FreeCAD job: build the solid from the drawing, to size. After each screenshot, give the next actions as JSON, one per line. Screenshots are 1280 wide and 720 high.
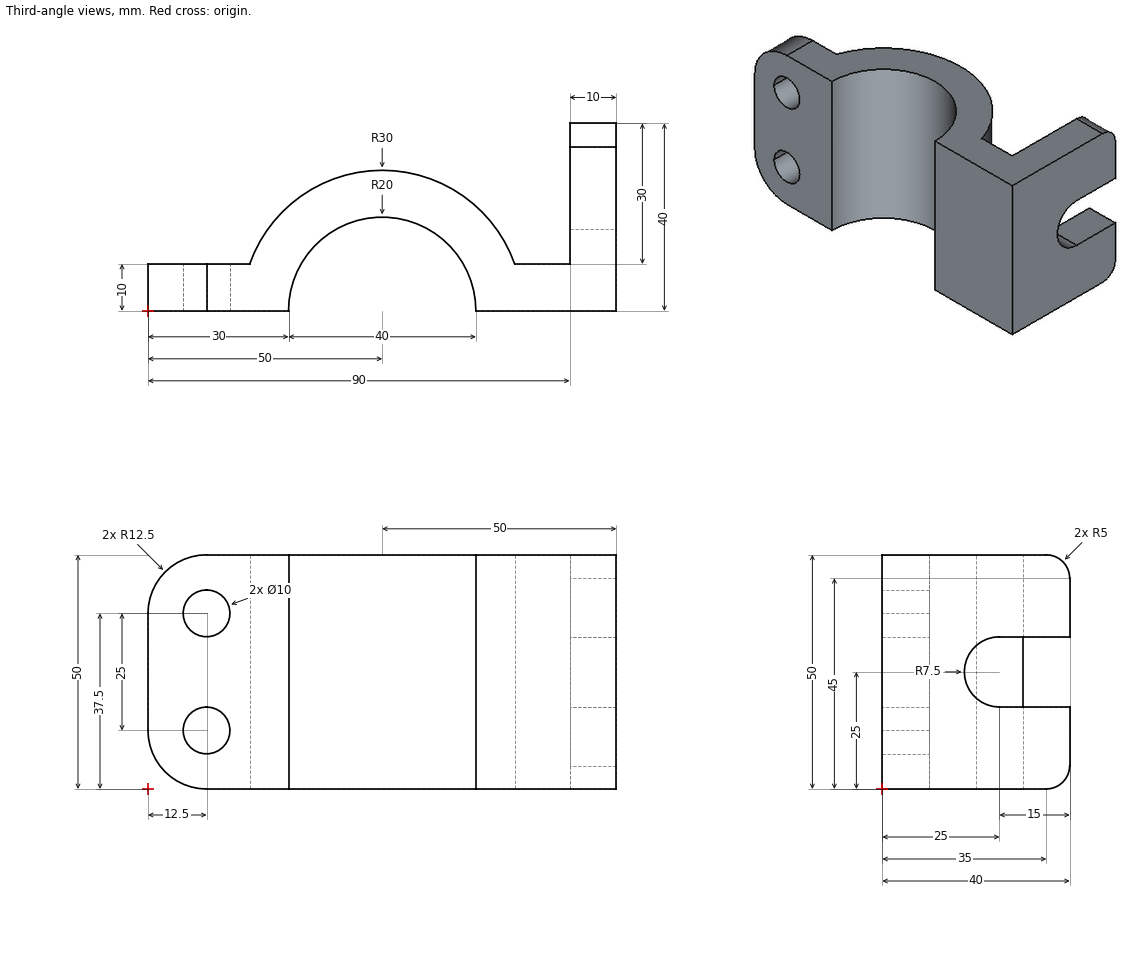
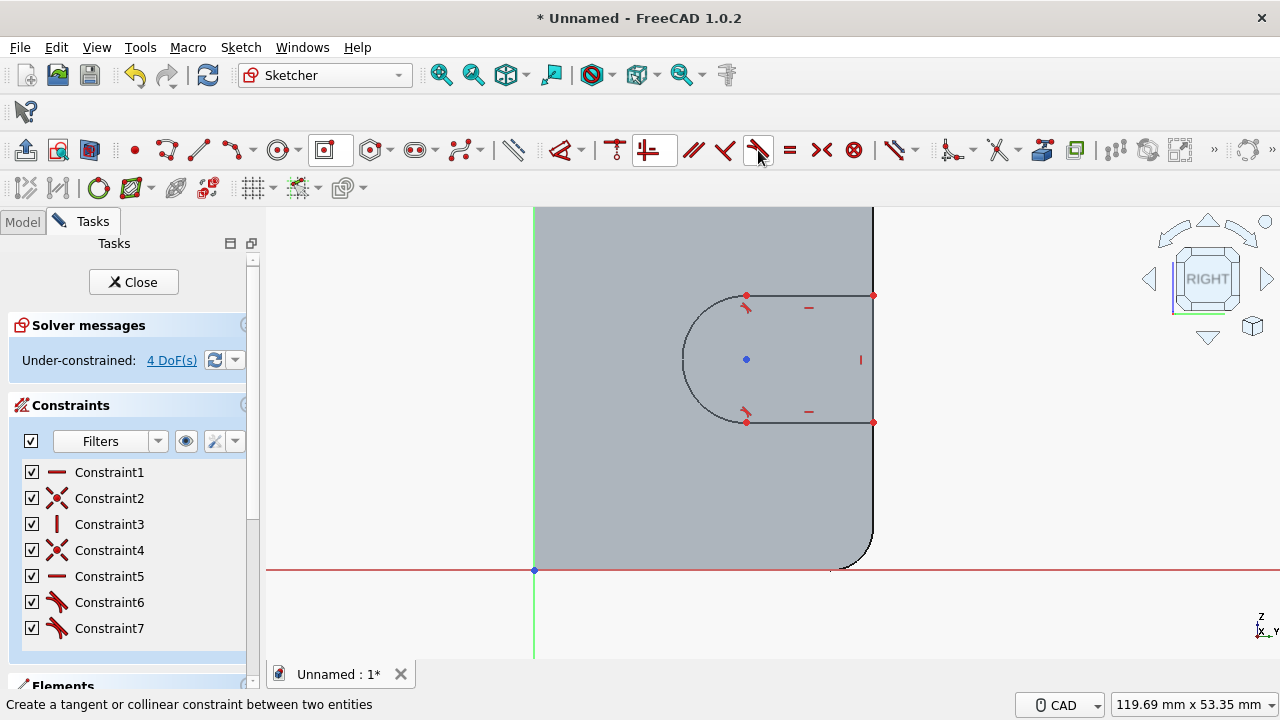
{"action": "left_click", "coordinate": [560, 150]}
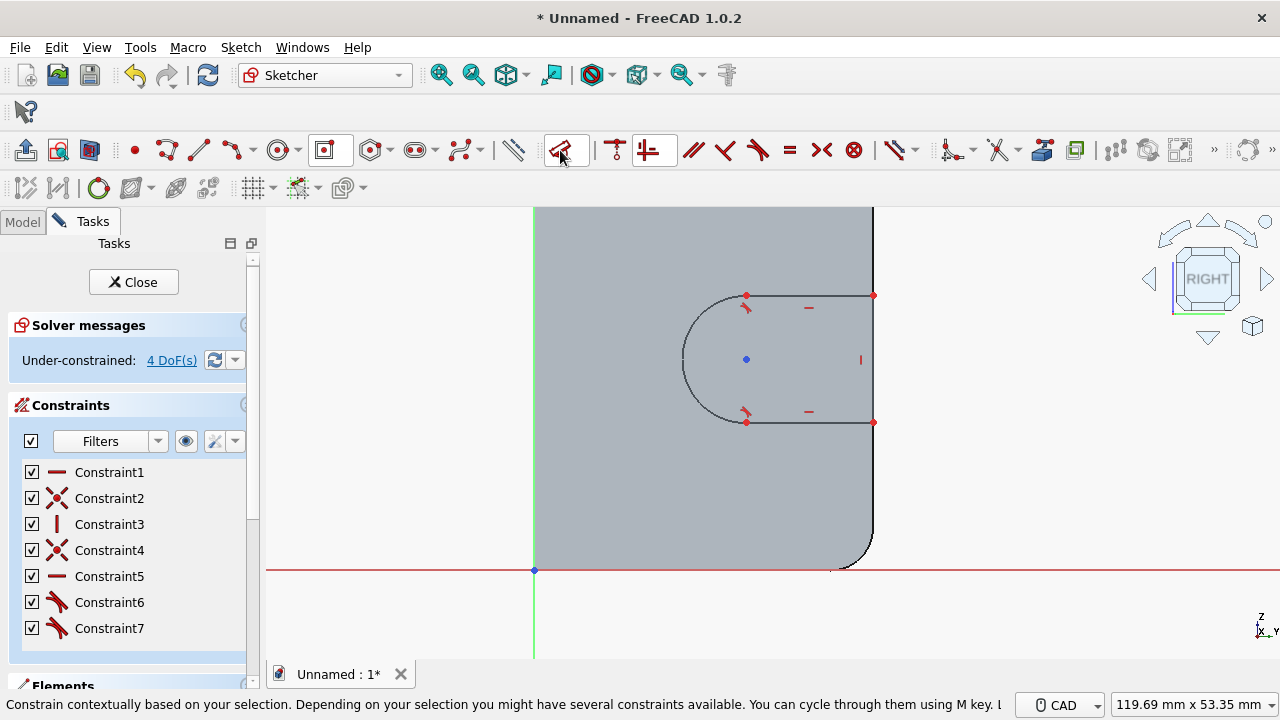
{"action": "left_click", "coordinate": [695, 322]}
{"action": "left_click", "coordinate": [669, 303]}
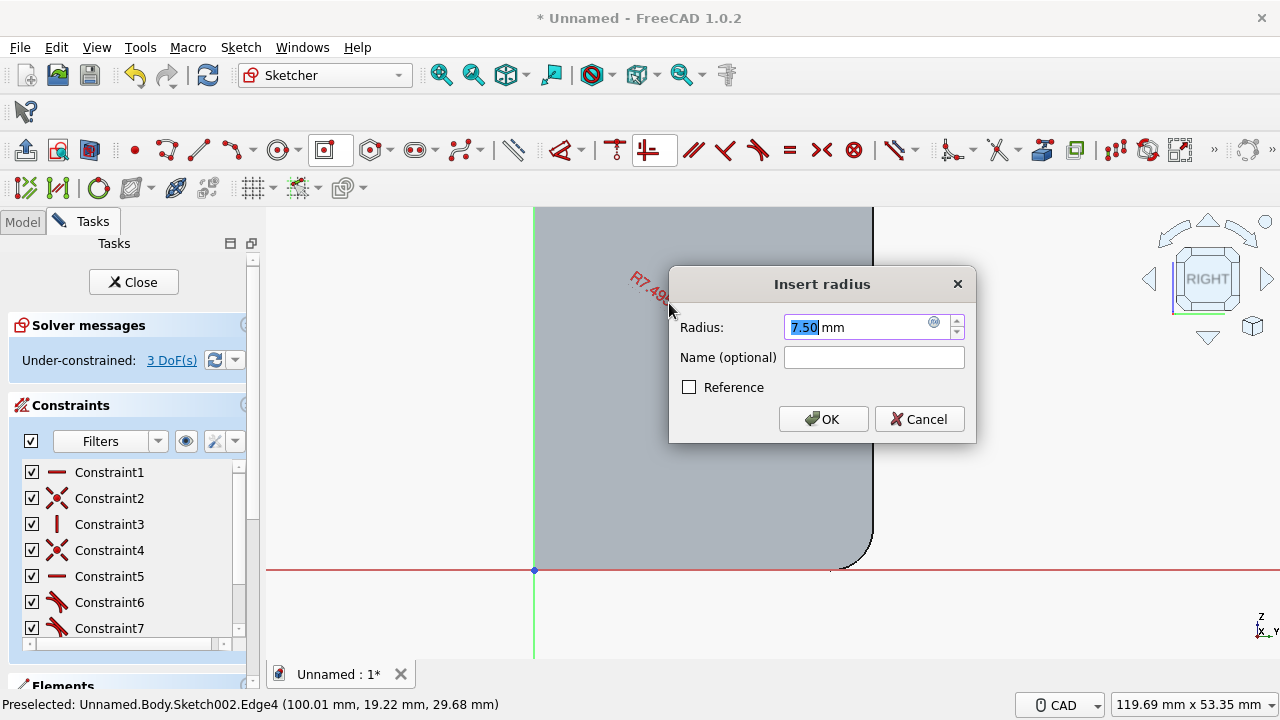
{"action": "type", "text": "7.5"}
{"action": "key", "text": "Return"}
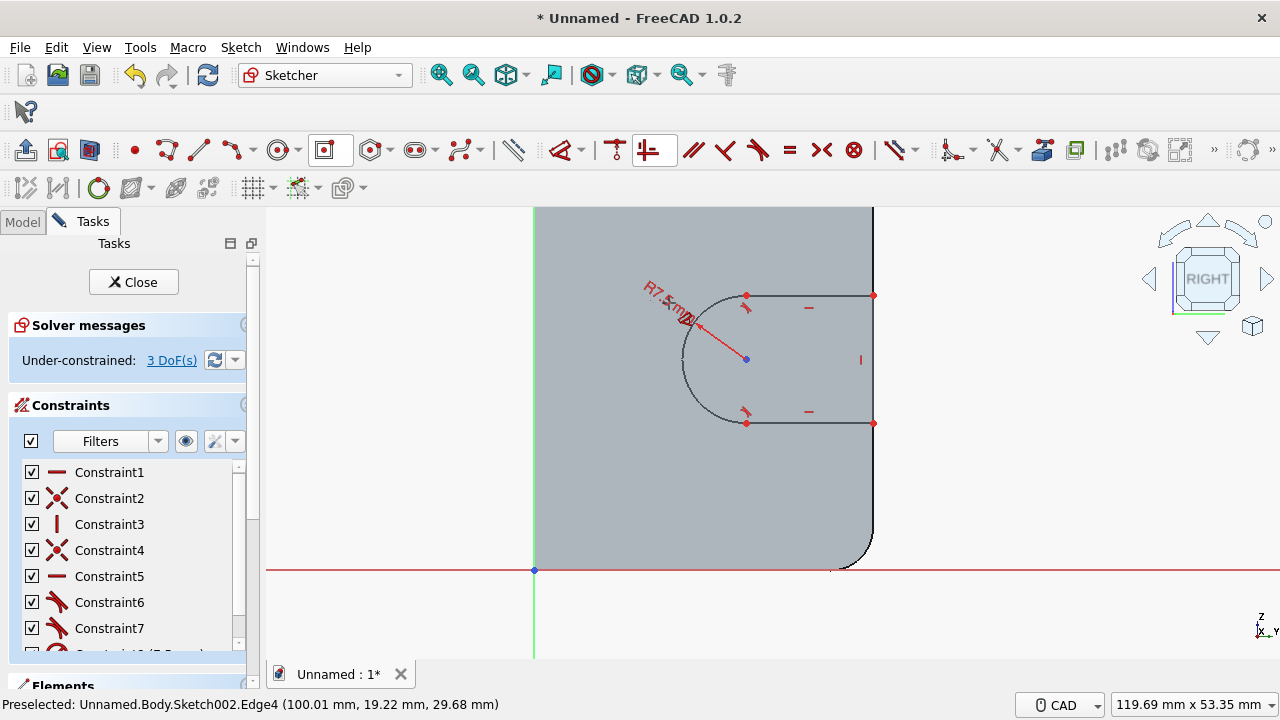
{"action": "left_click", "coordinate": [784, 423]}
{"action": "left_click", "coordinate": [810, 389]}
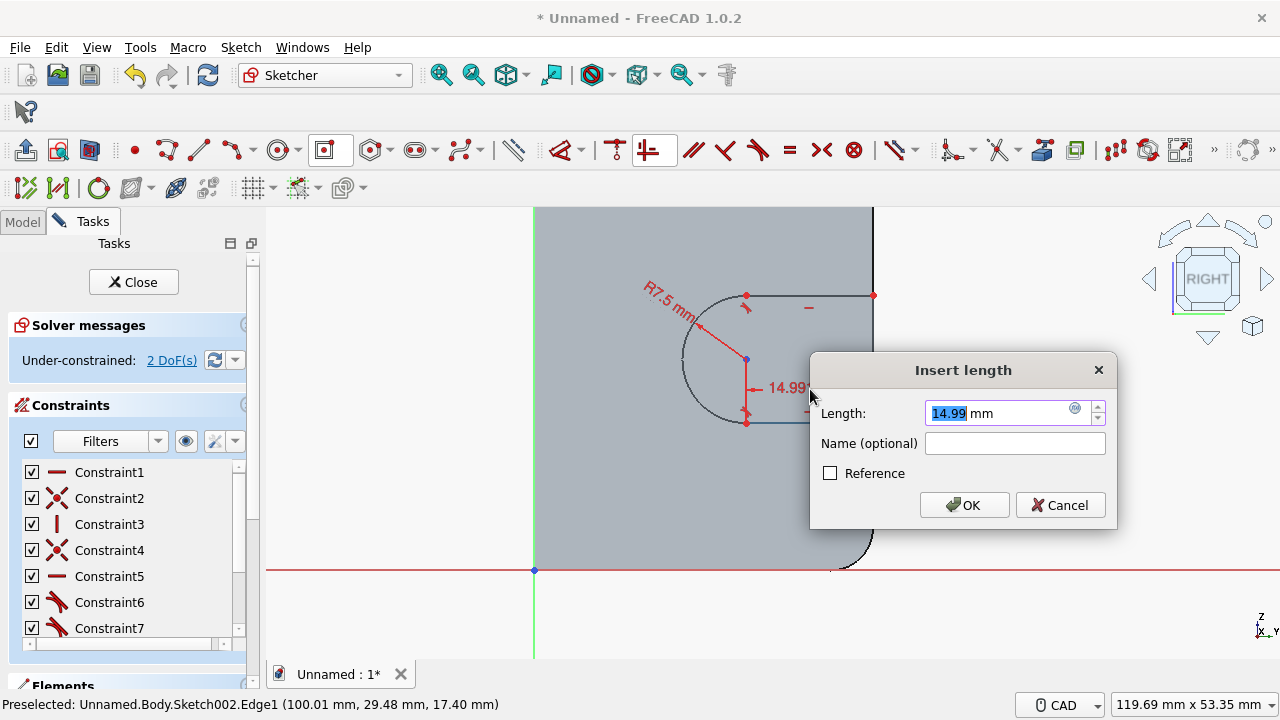
{"action": "type", "text": "15"}
{"action": "key", "text": "Return"}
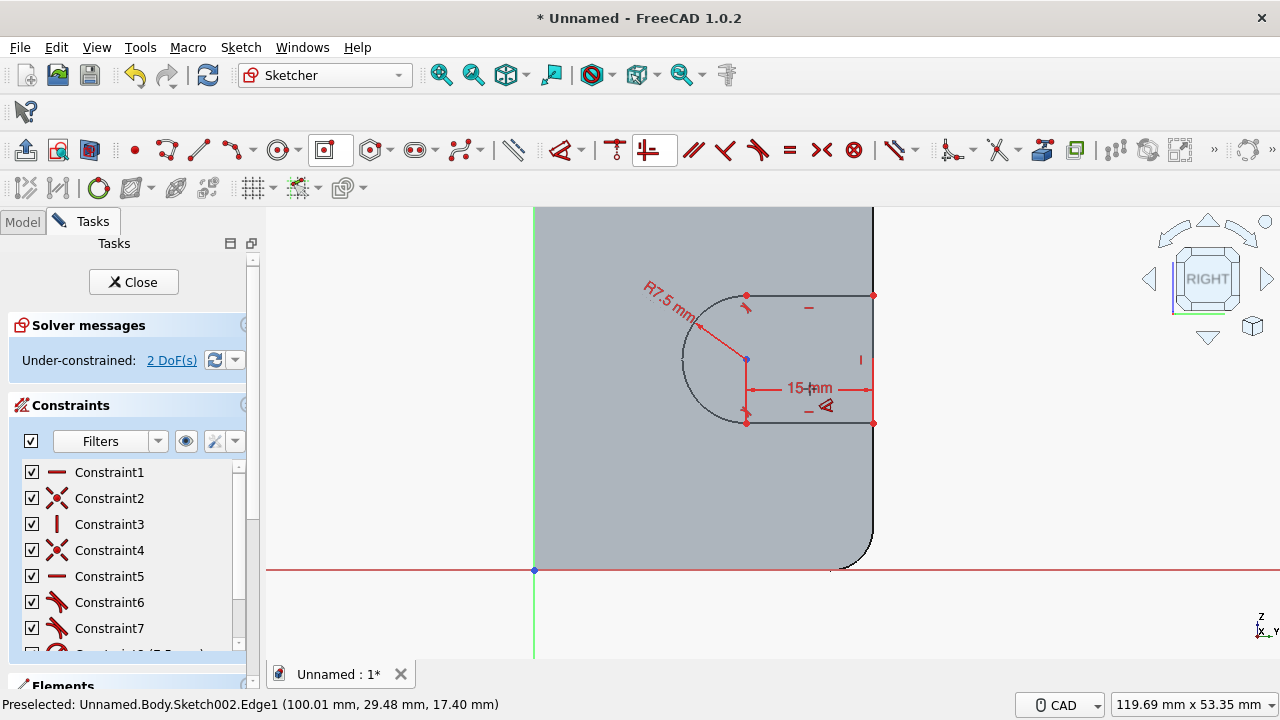
{"action": "left_click", "coordinate": [746, 423]}
{"action": "left_click", "coordinate": [640, 604]}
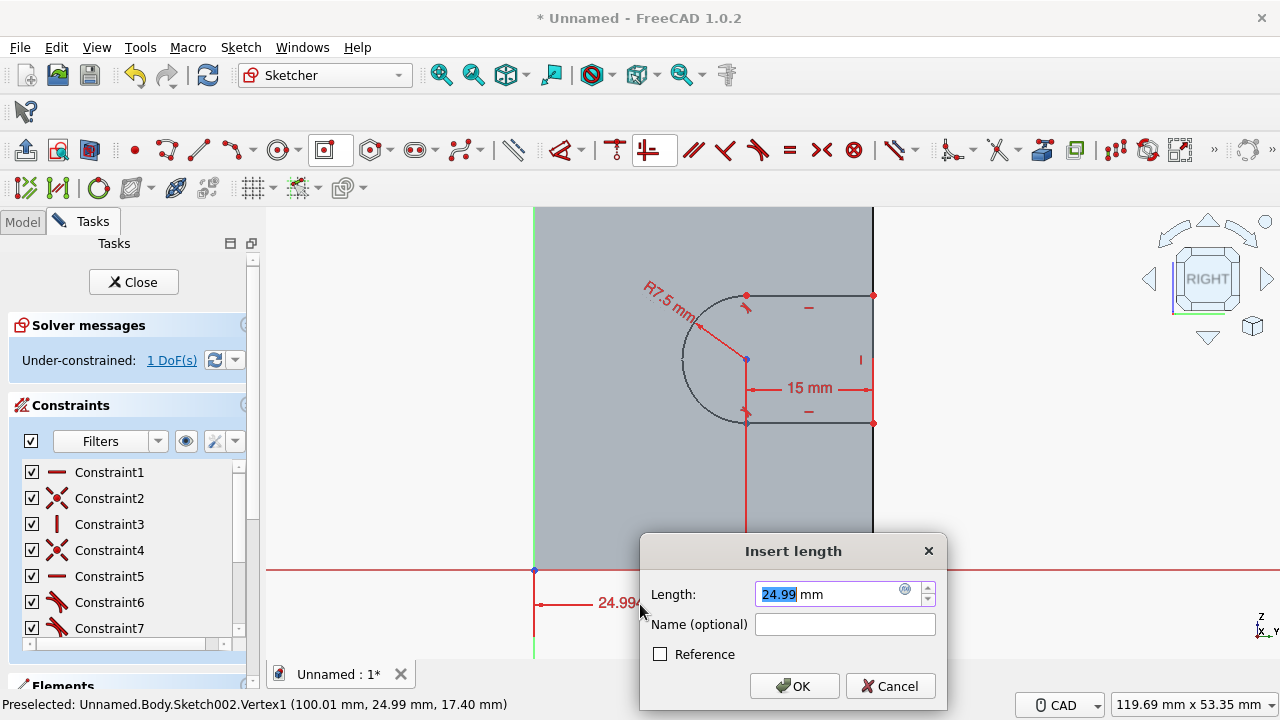
{"action": "type", "text": "25"}
{"action": "key", "text": "Return"}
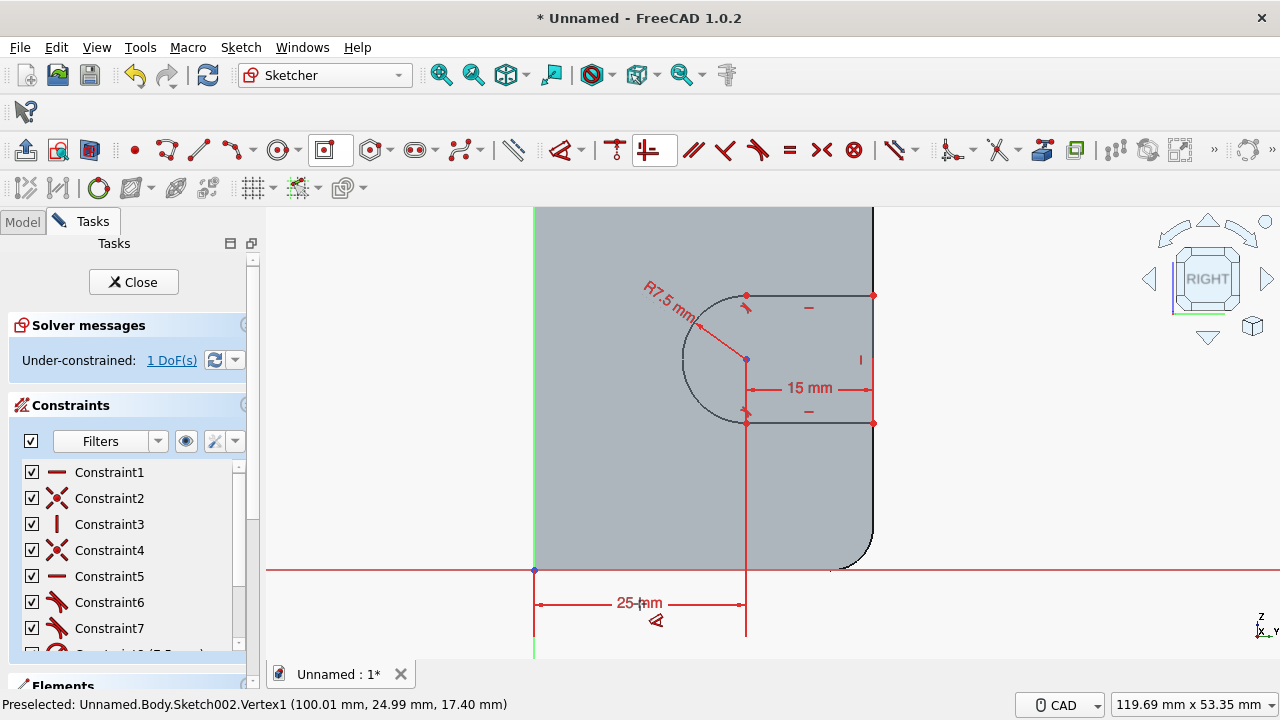
{"action": "left_click", "coordinate": [746, 360]}
{"action": "left_click", "coordinate": [500, 465]}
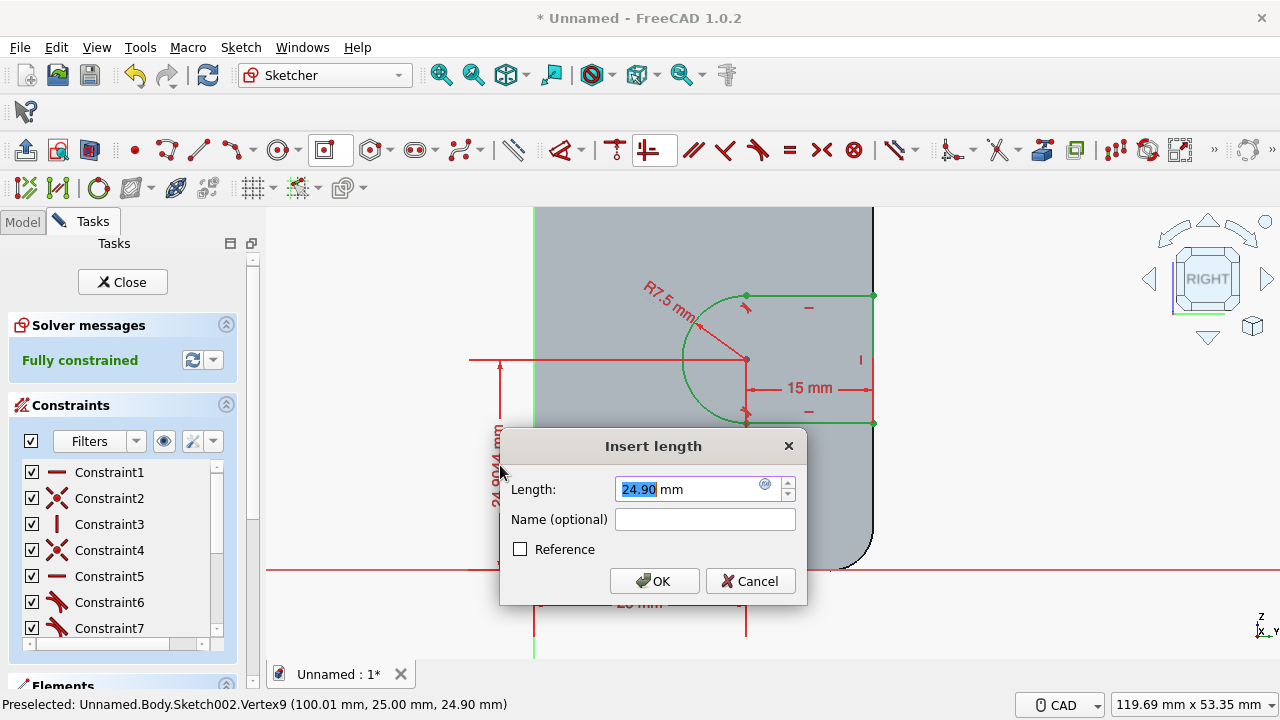
{"action": "type", "text": "25"}
{"action": "key", "text": "Return"}
{"action": "key", "text": "Escape"}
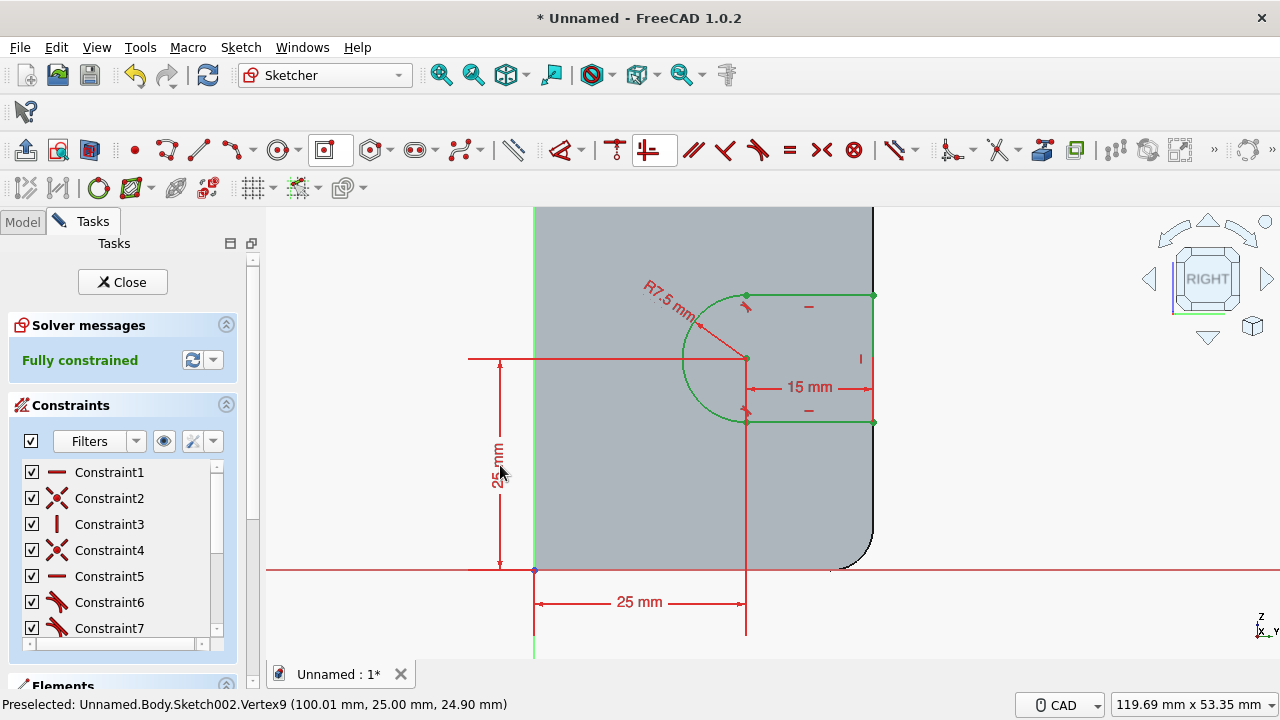
{"action": "left_click", "coordinate": [123, 282]}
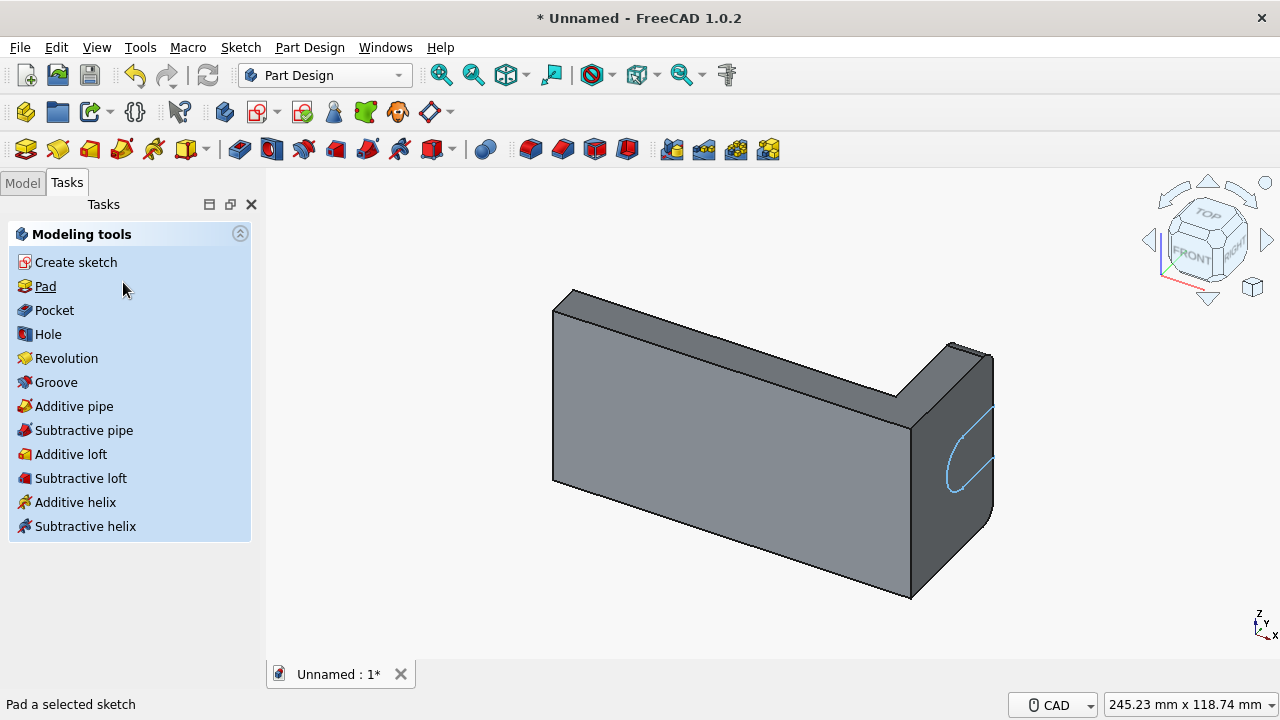
{"action": "left_click", "coordinate": [240, 150]}